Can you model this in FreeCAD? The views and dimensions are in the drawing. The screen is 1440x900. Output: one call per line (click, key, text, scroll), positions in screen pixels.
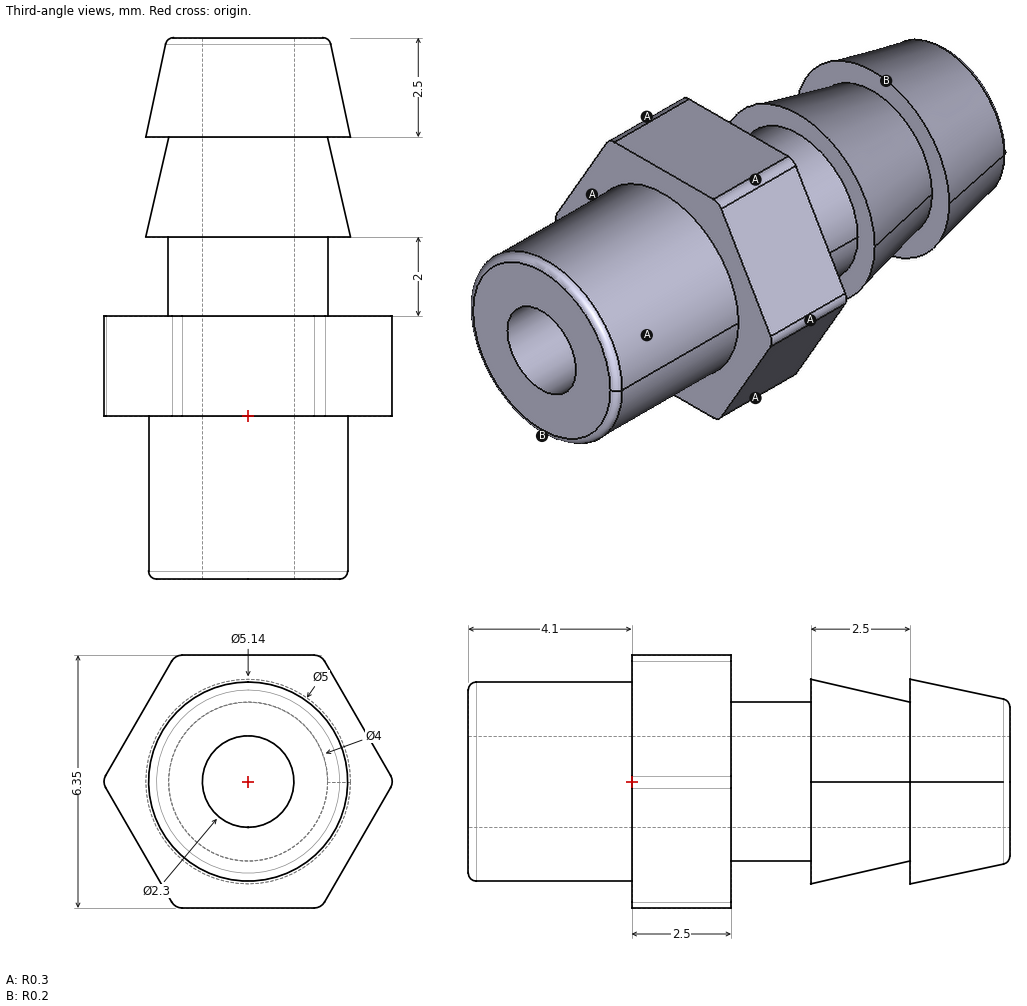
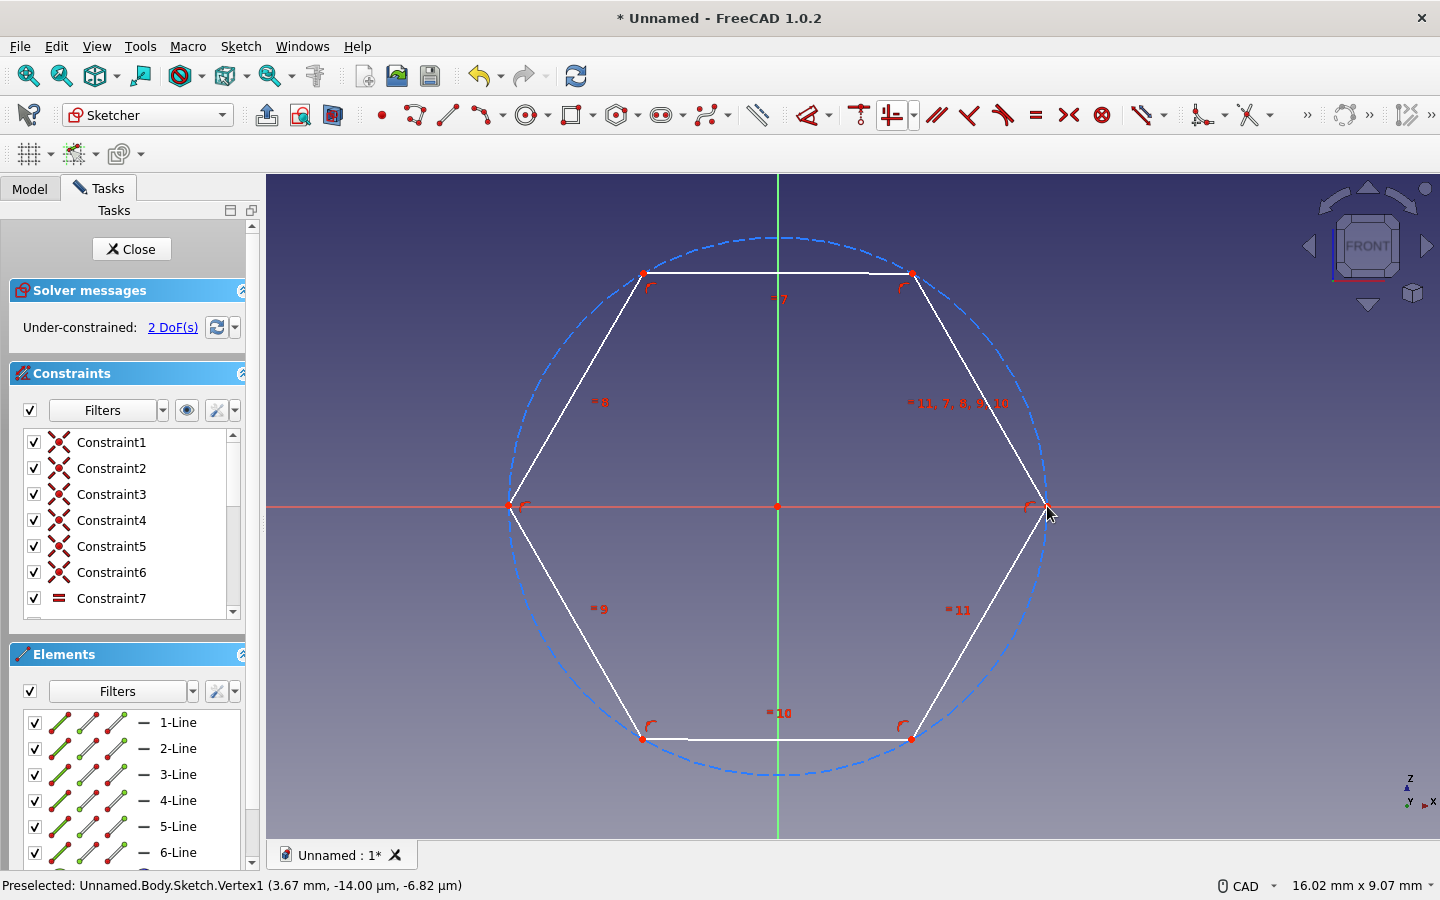
click(832, 273)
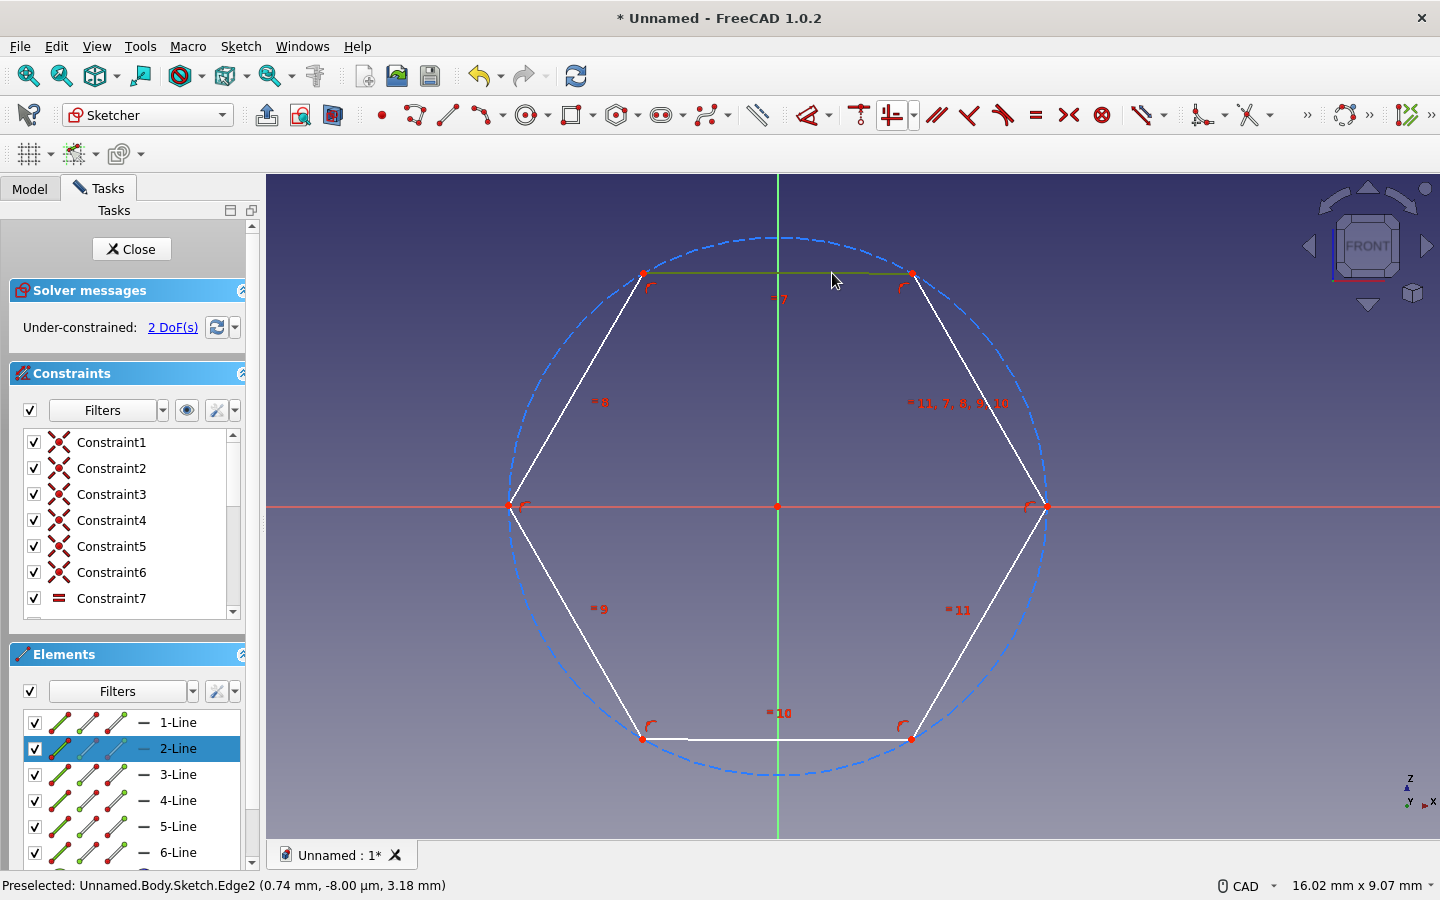
key(h)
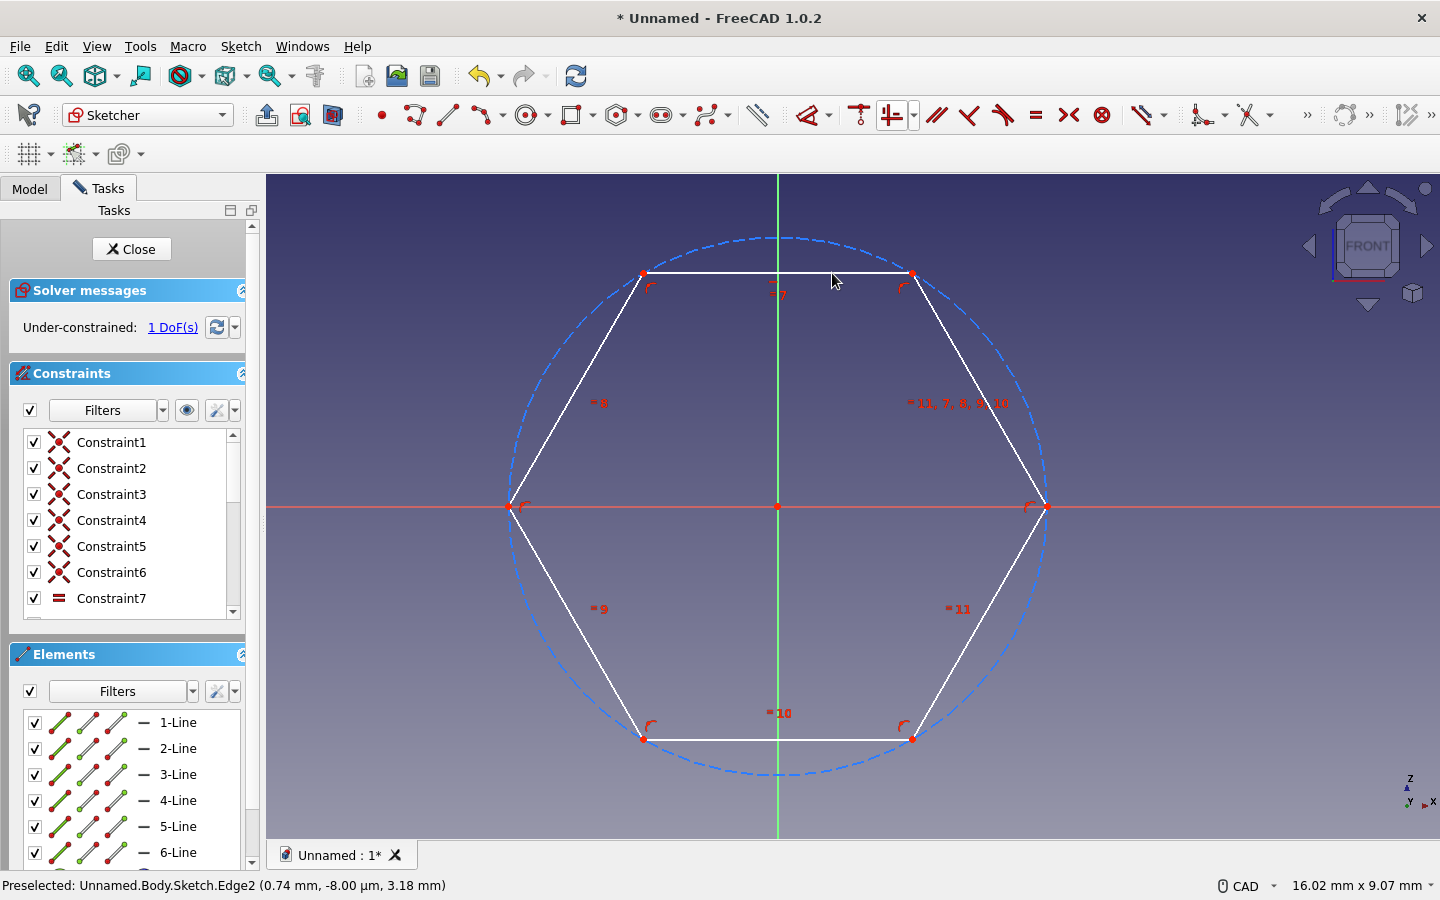
click(806, 116)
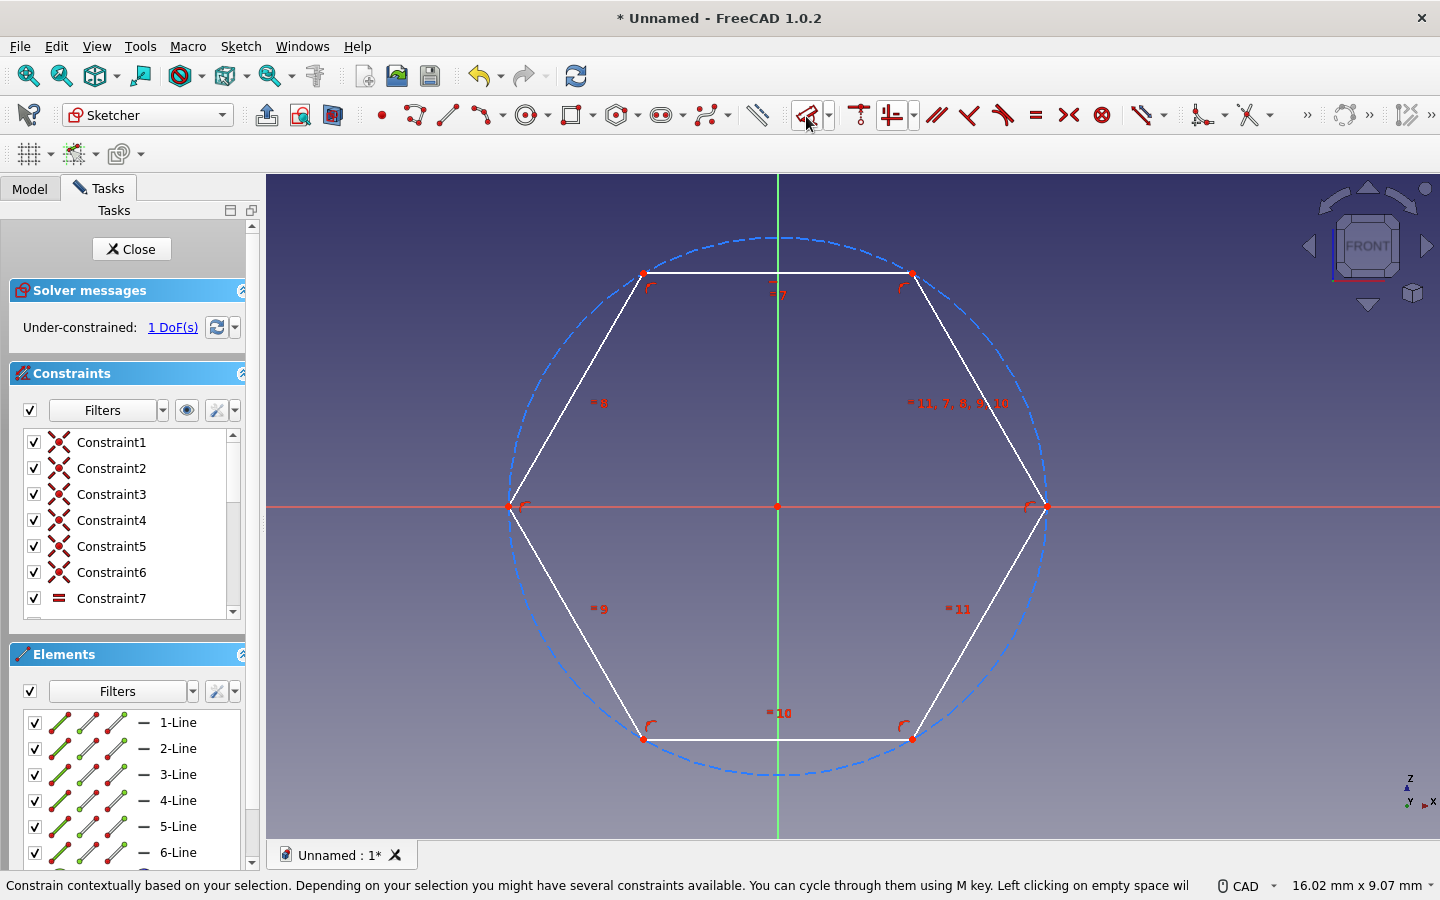
click(643, 740)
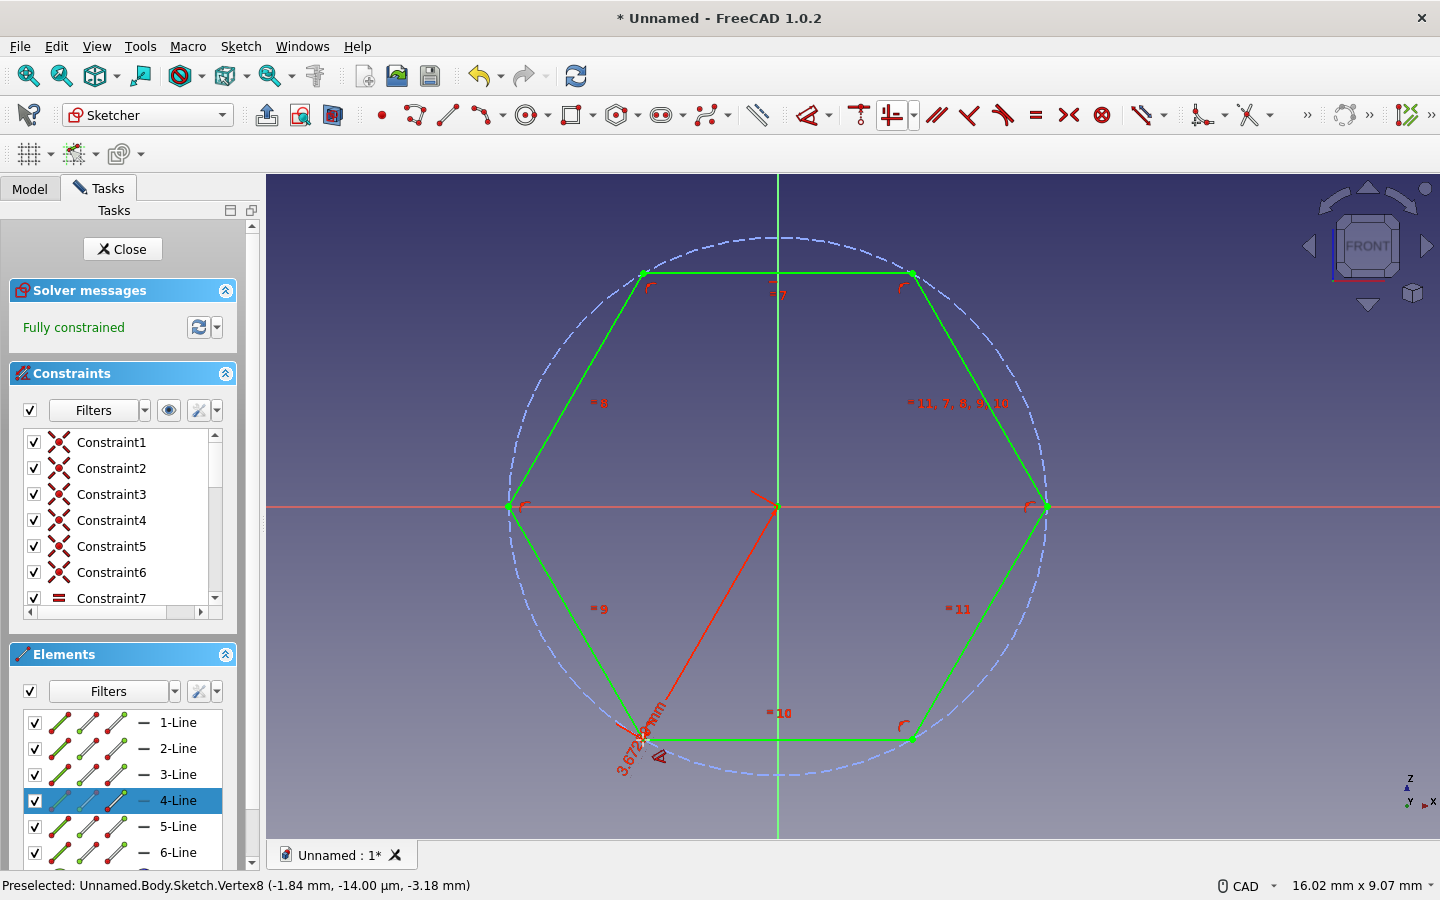
click(912, 273)
click(946, 399)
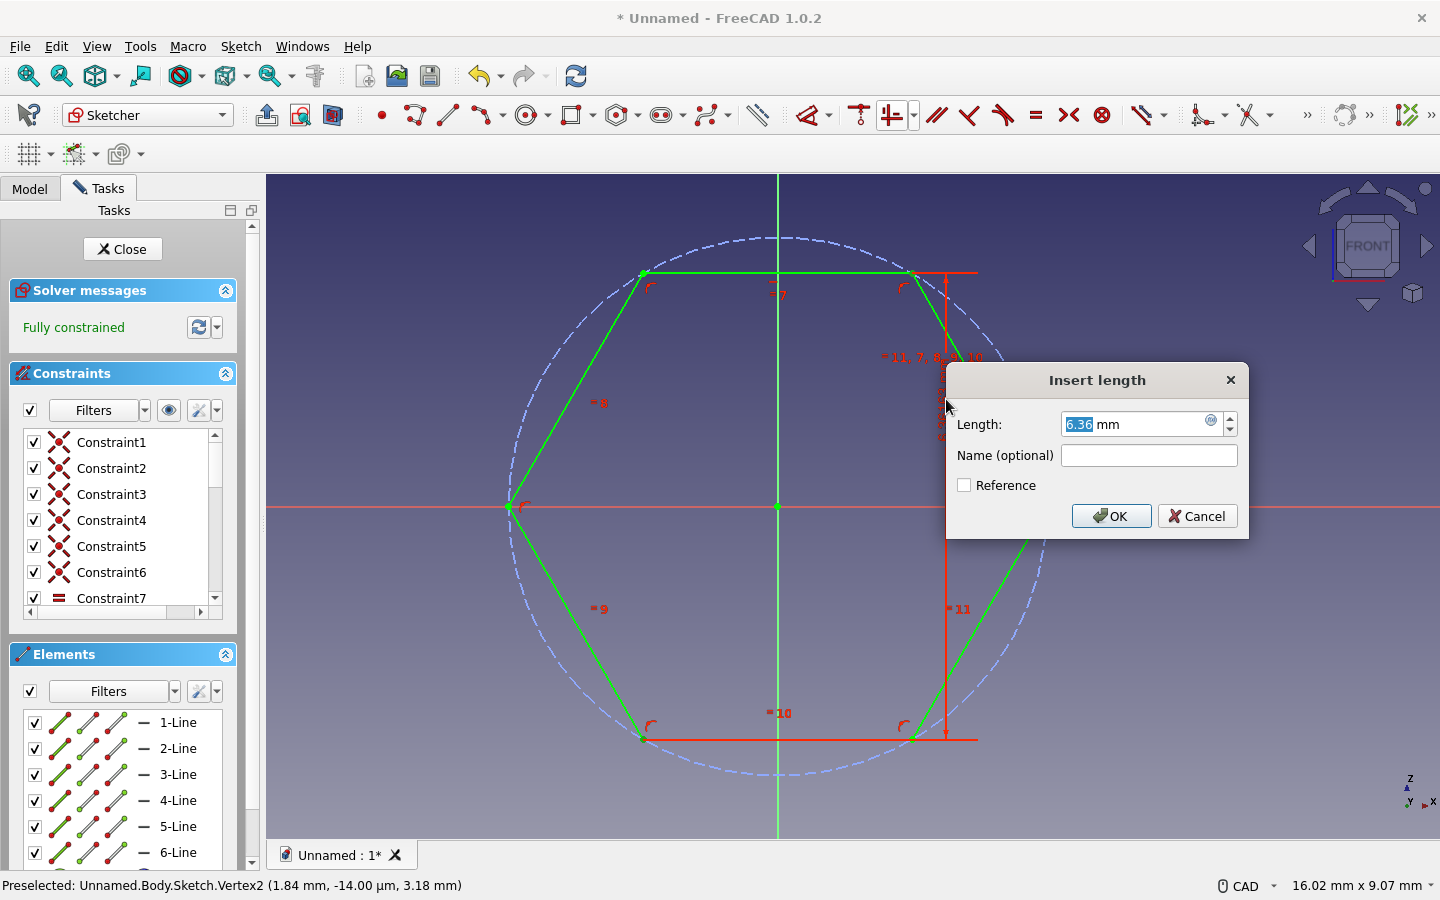
text(6.35)
key(Return)
key(Escape)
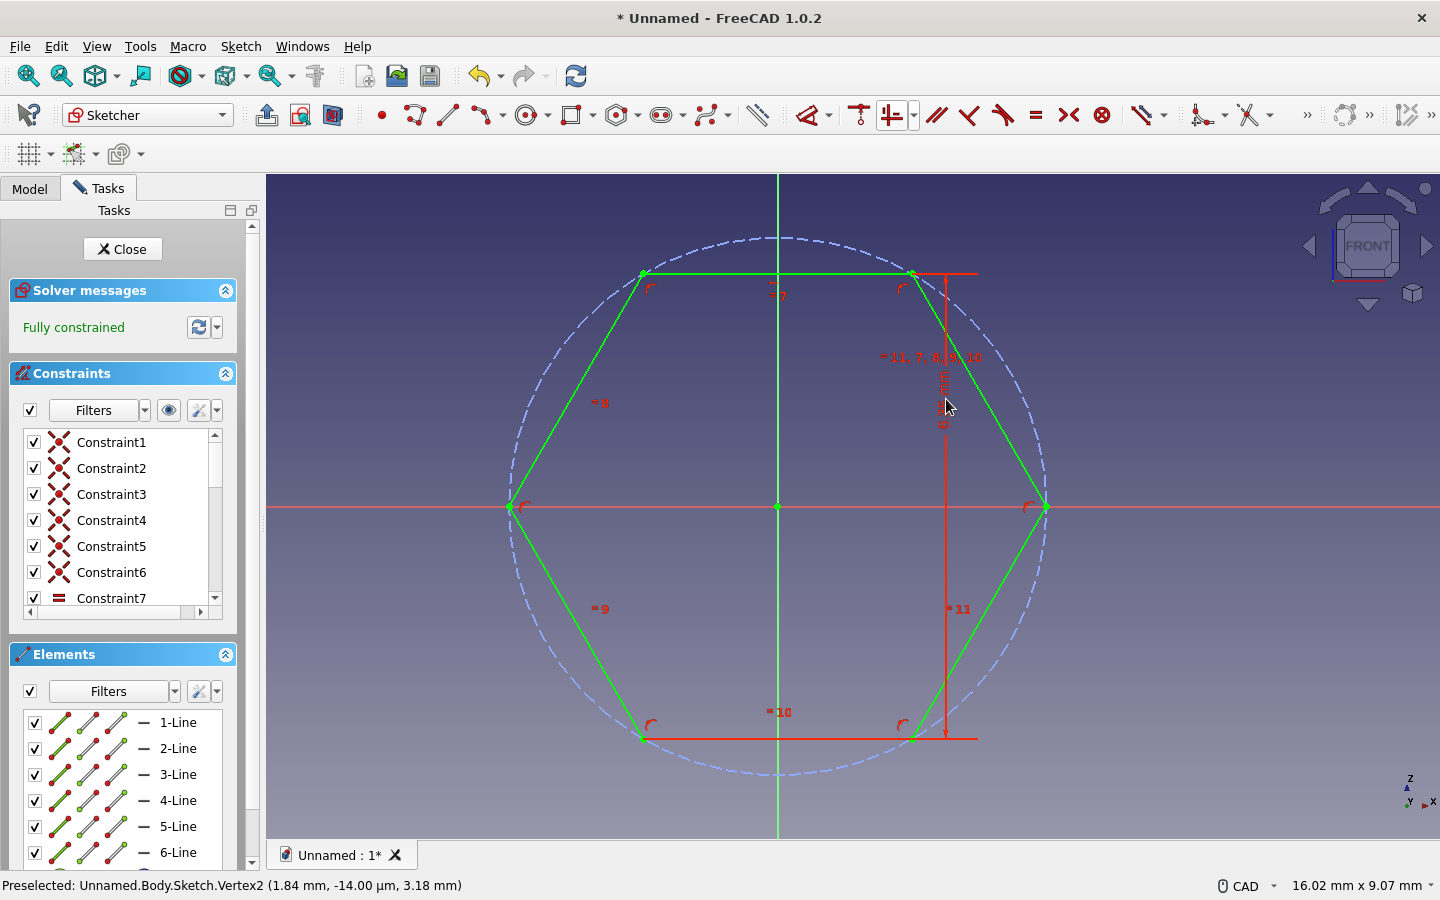
click(123, 249)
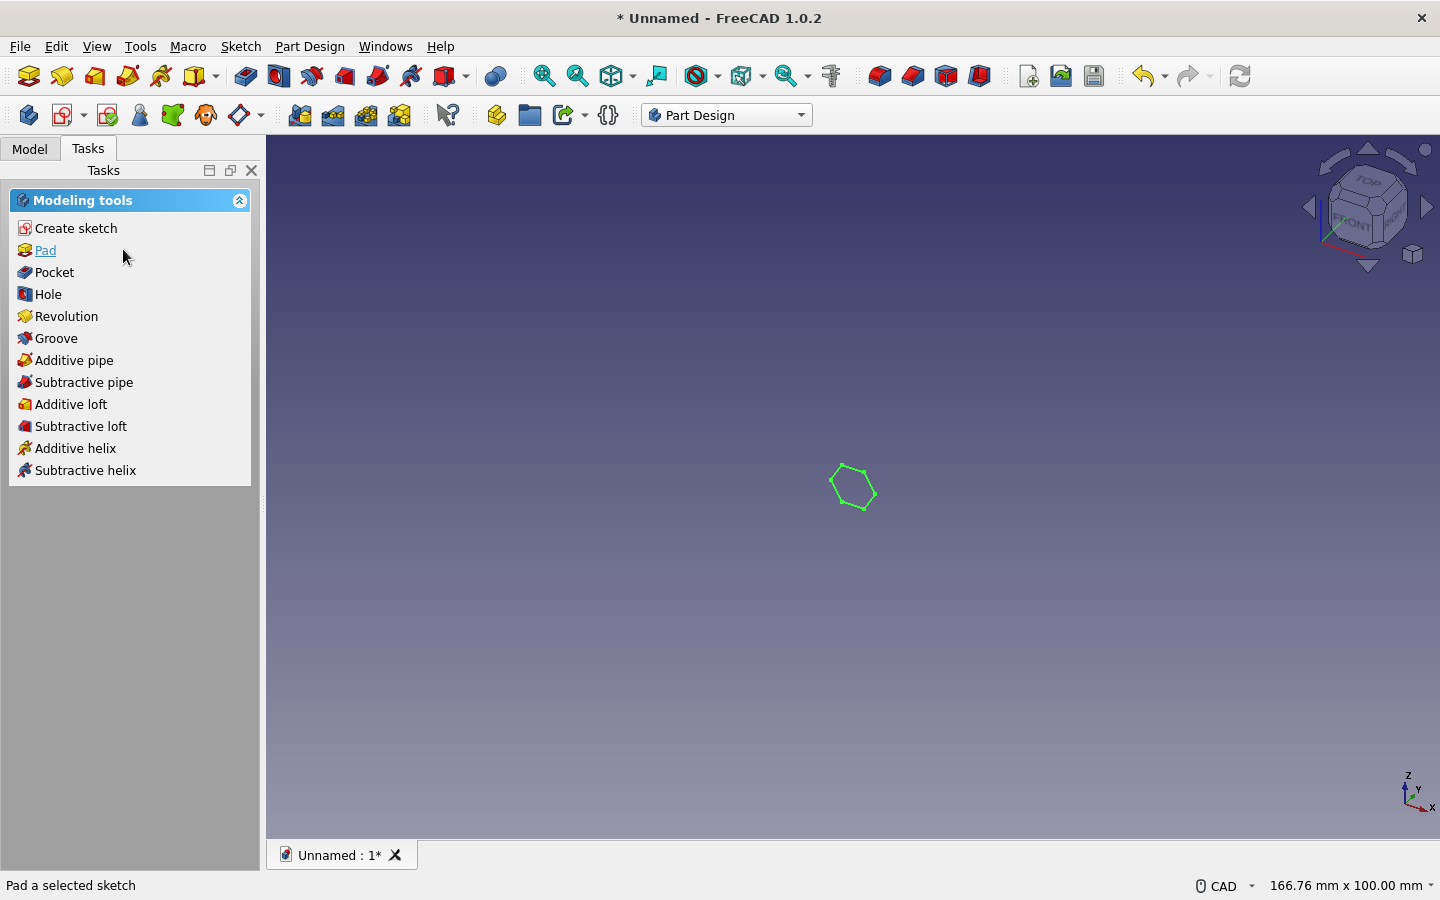
click(29, 76)